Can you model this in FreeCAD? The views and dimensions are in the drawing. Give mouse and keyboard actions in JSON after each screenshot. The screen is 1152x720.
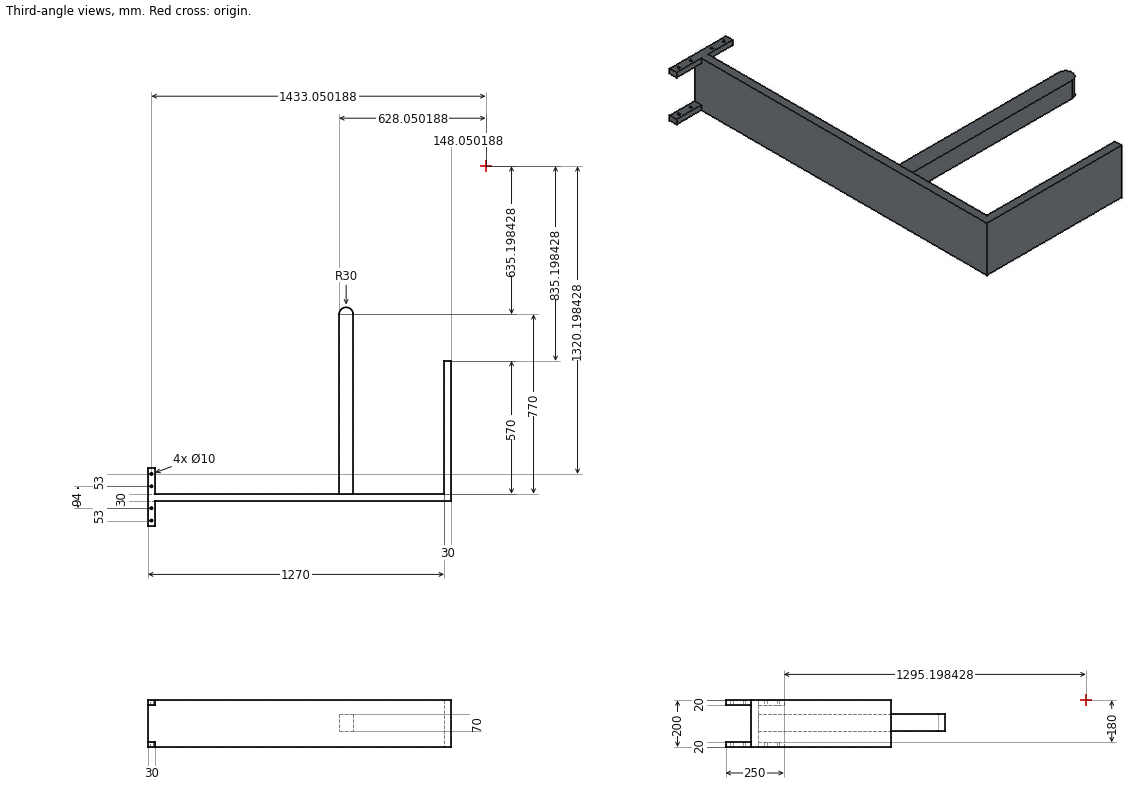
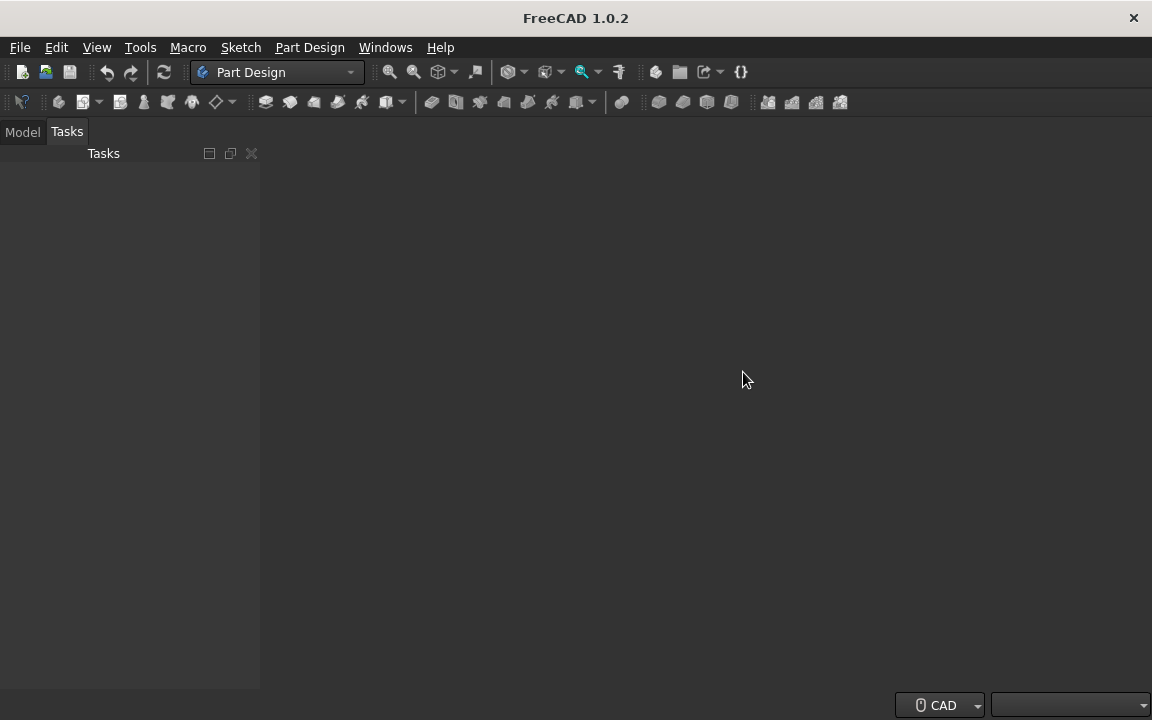
{"action": "left_click", "coordinate": [22, 72]}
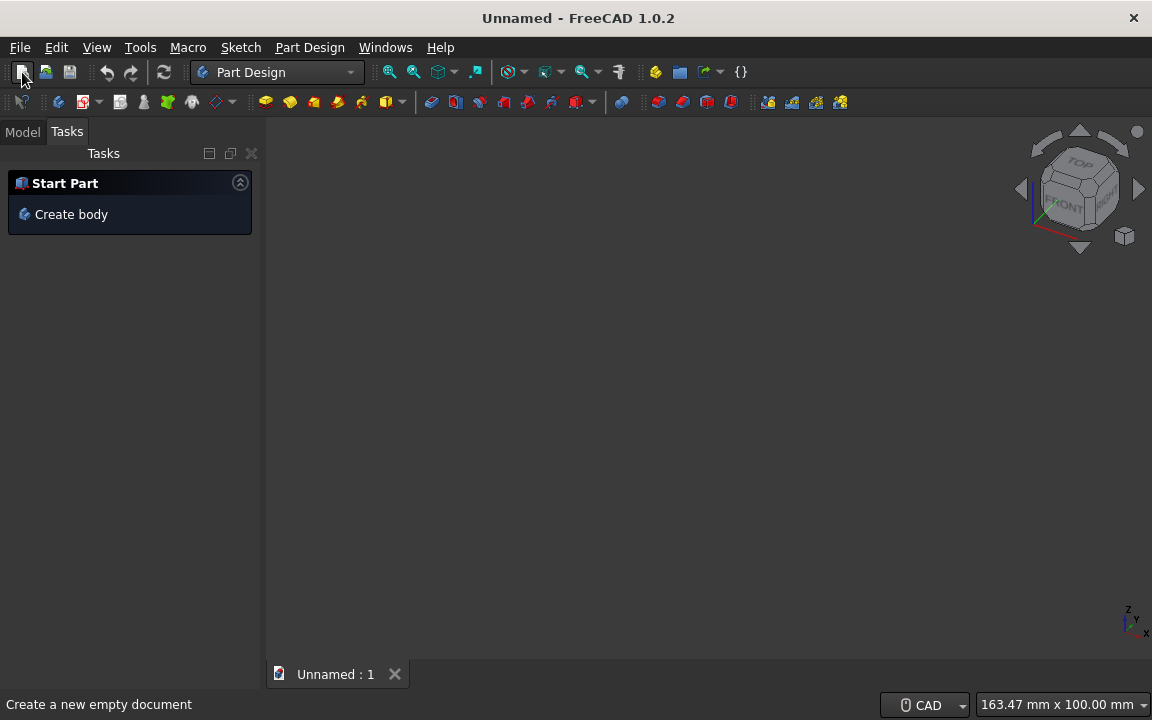
{"action": "left_click", "coordinate": [84, 102]}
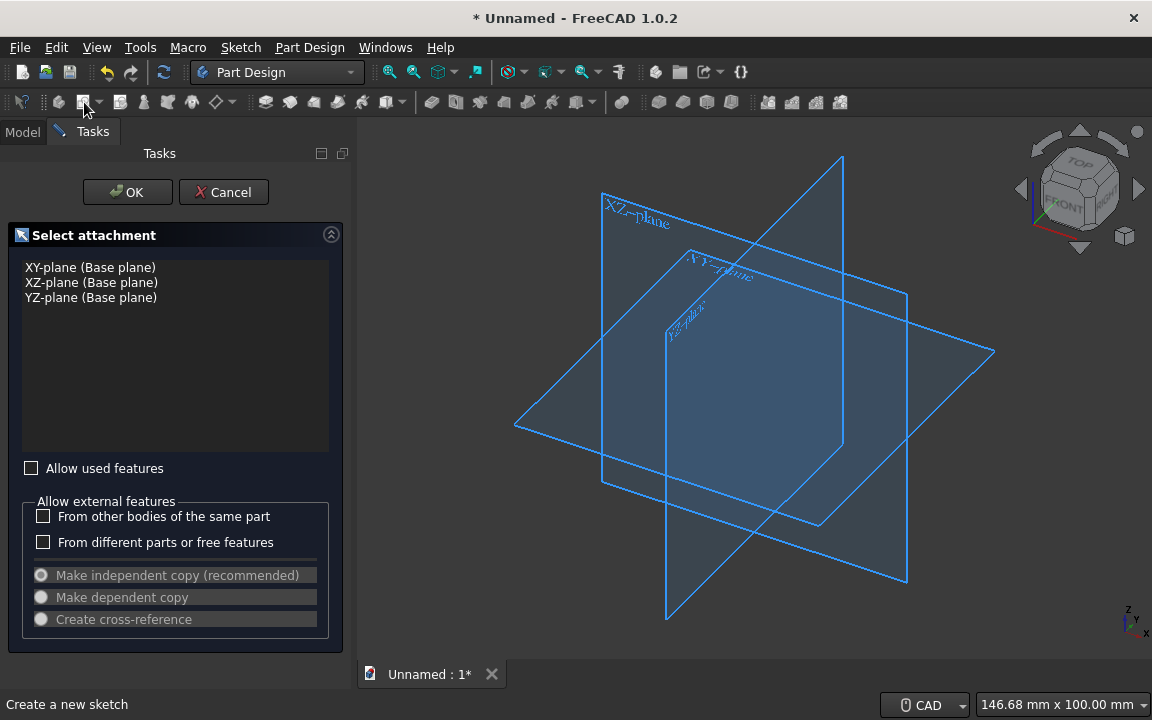
{"action": "left_click", "coordinate": [82, 268]}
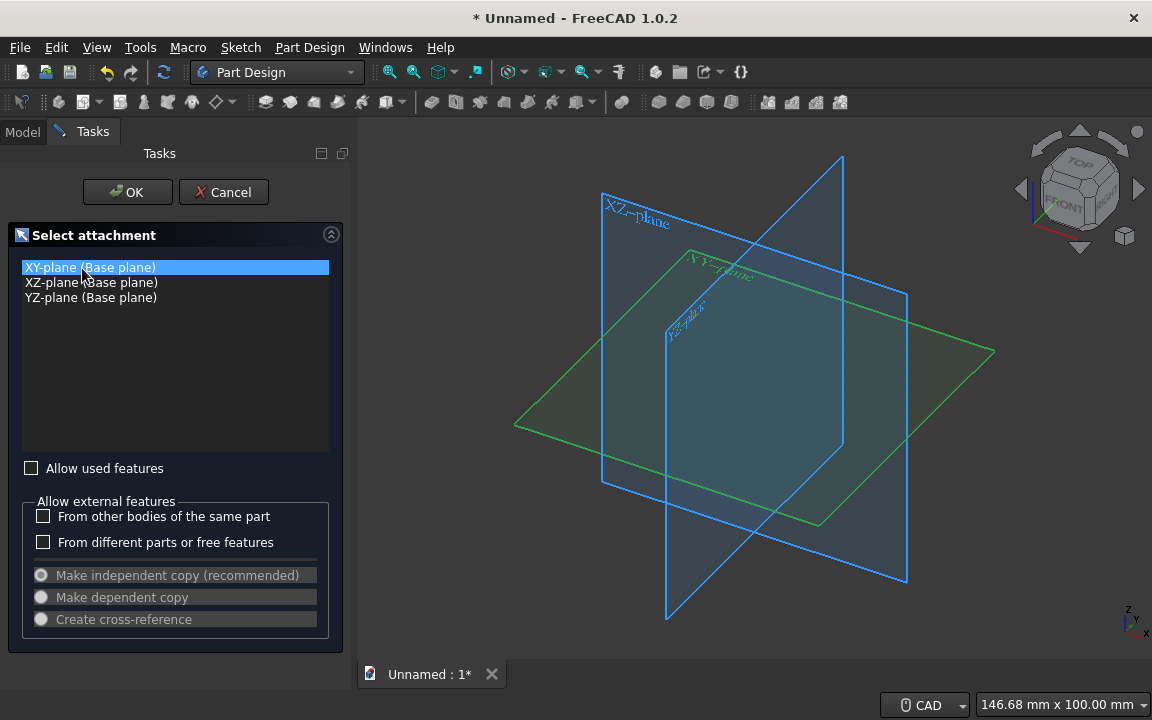
{"action": "left_click", "coordinate": [128, 192]}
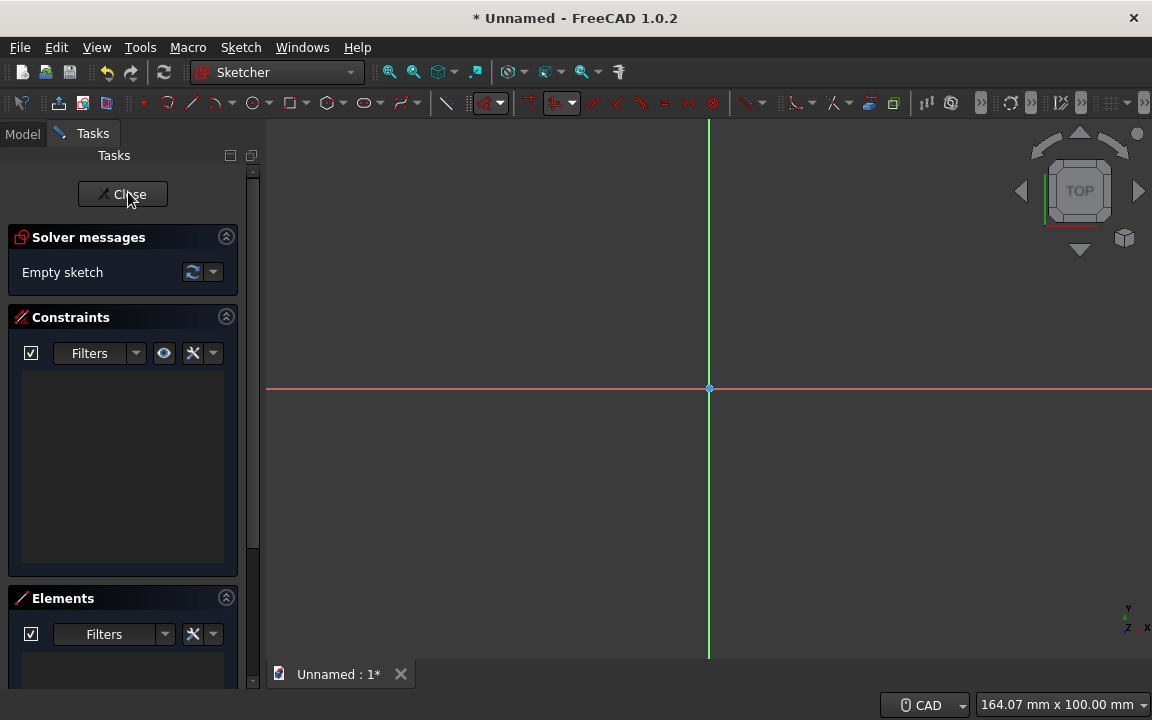
{"action": "scroll", "coordinate": [842, 186], "scroll_direction": "down", "scroll_amount": 15}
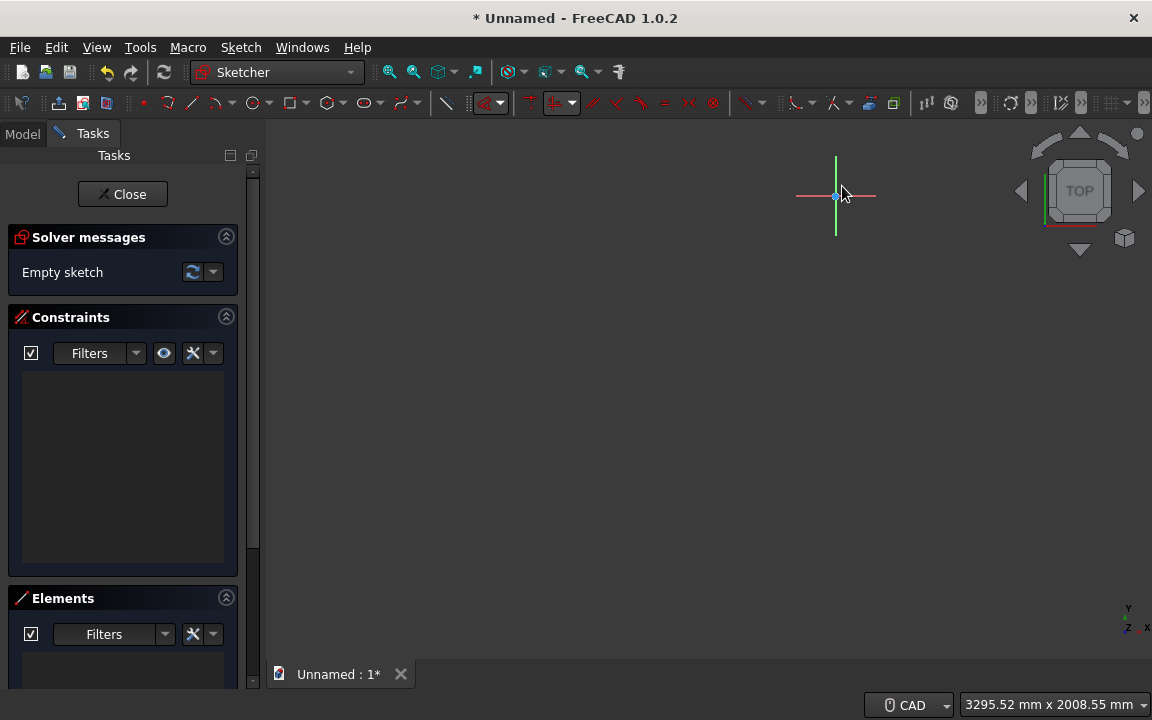
{"action": "left_click", "coordinate": [168, 104]}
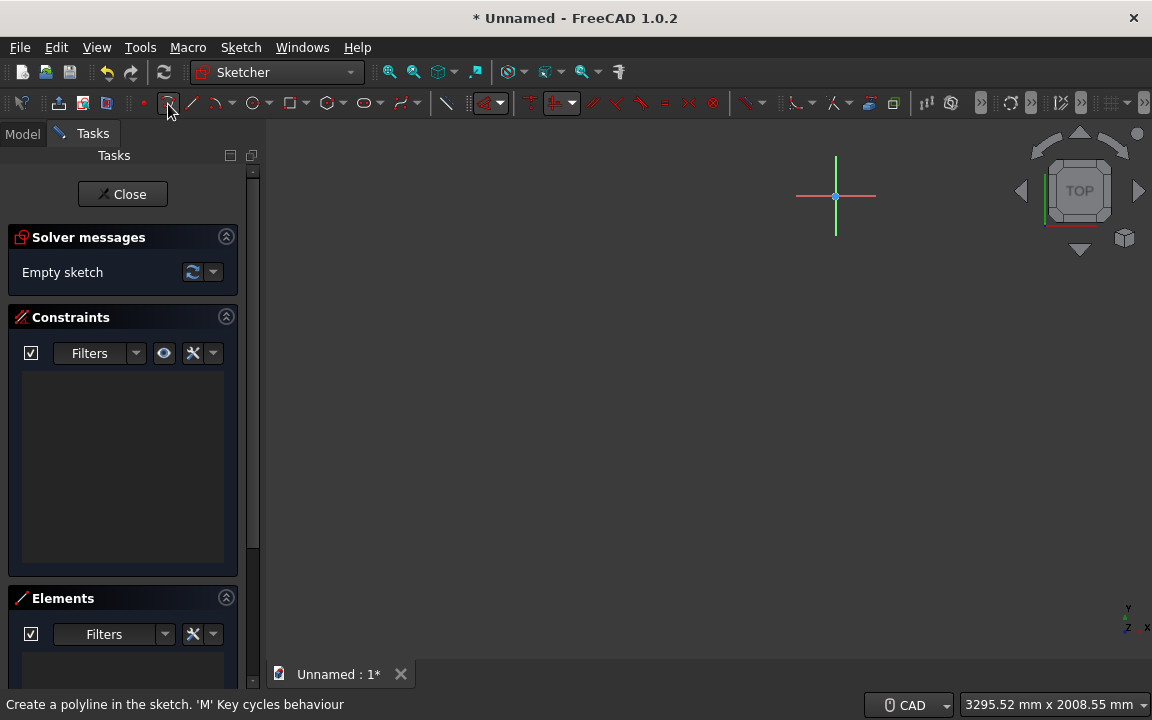
{"action": "left_click", "coordinate": [796, 421]}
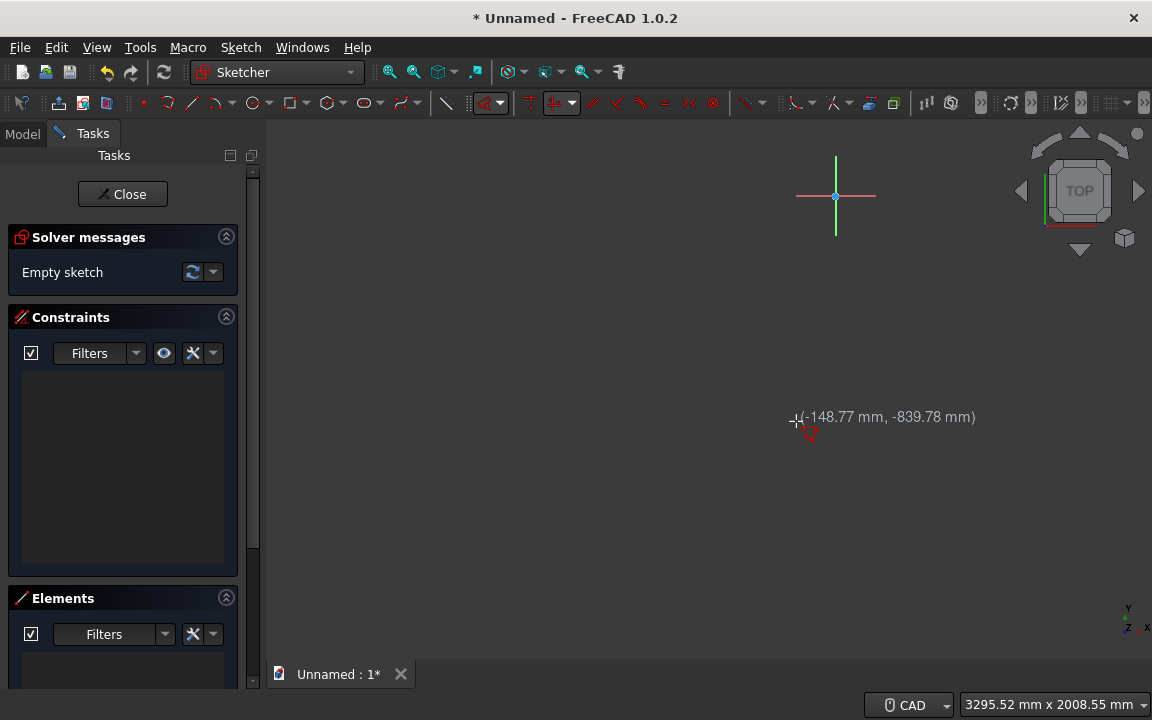
{"action": "scroll", "coordinate": [788, 421], "scroll_direction": "up", "scroll_amount": 4}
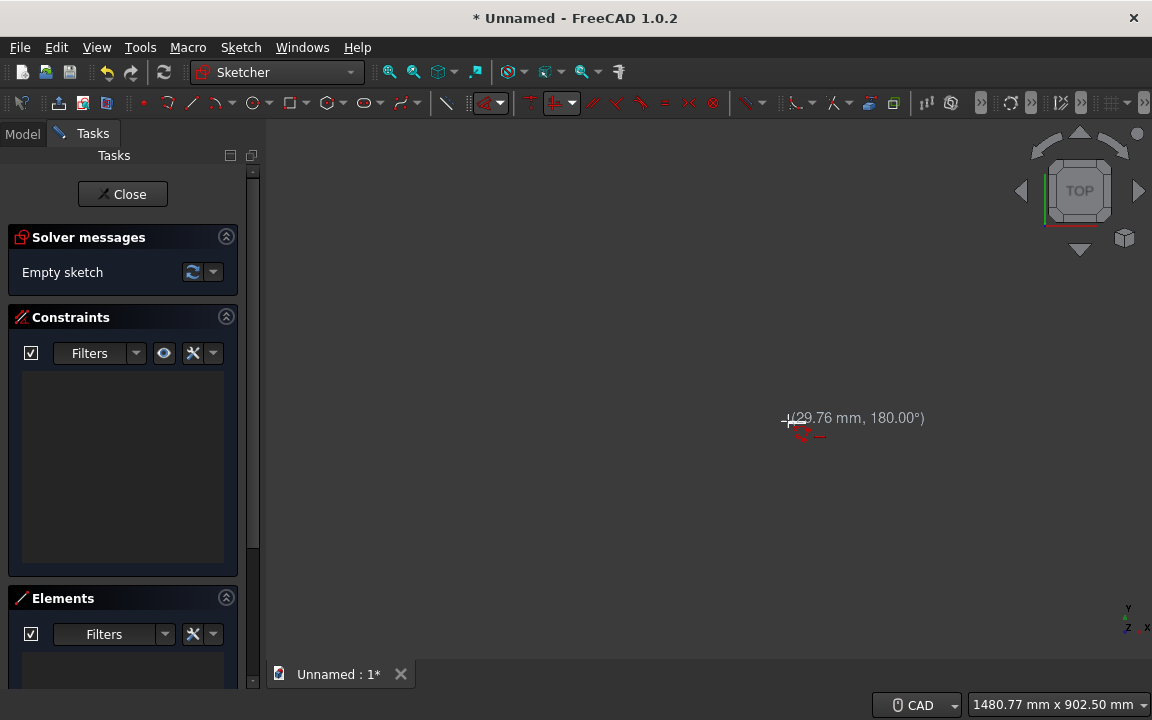
{"action": "left_click", "coordinate": [788, 420]}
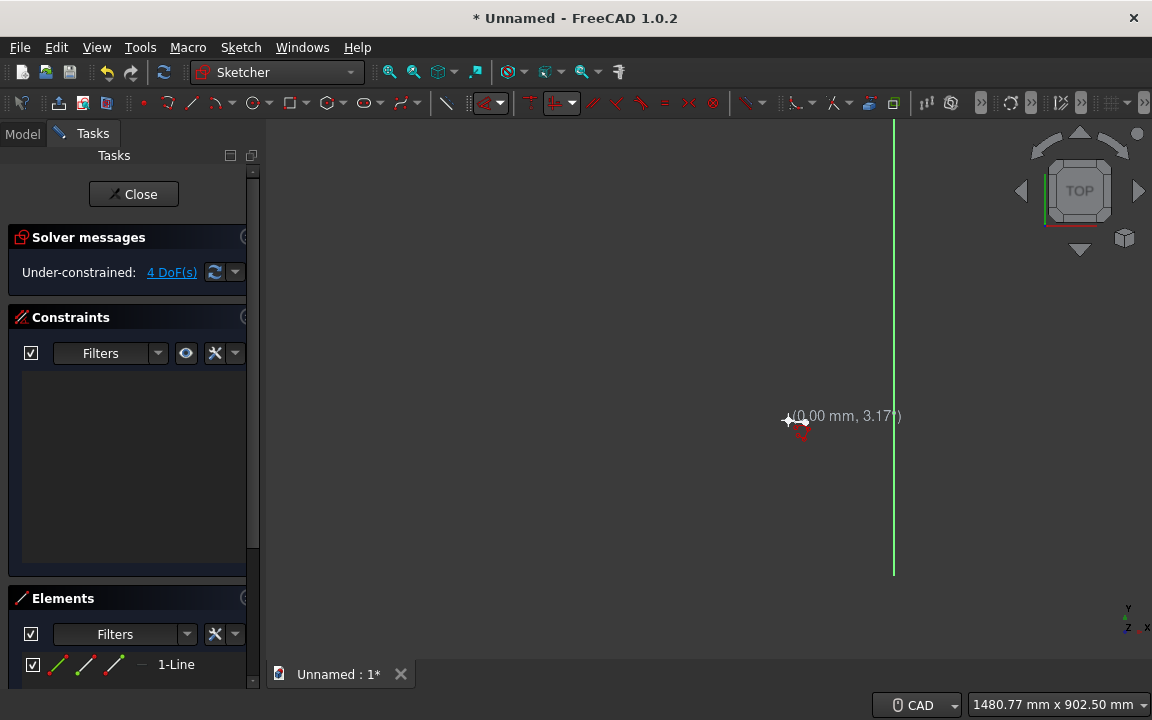
{"action": "scroll", "coordinate": [745, 412], "scroll_direction": "down", "scroll_amount": 5}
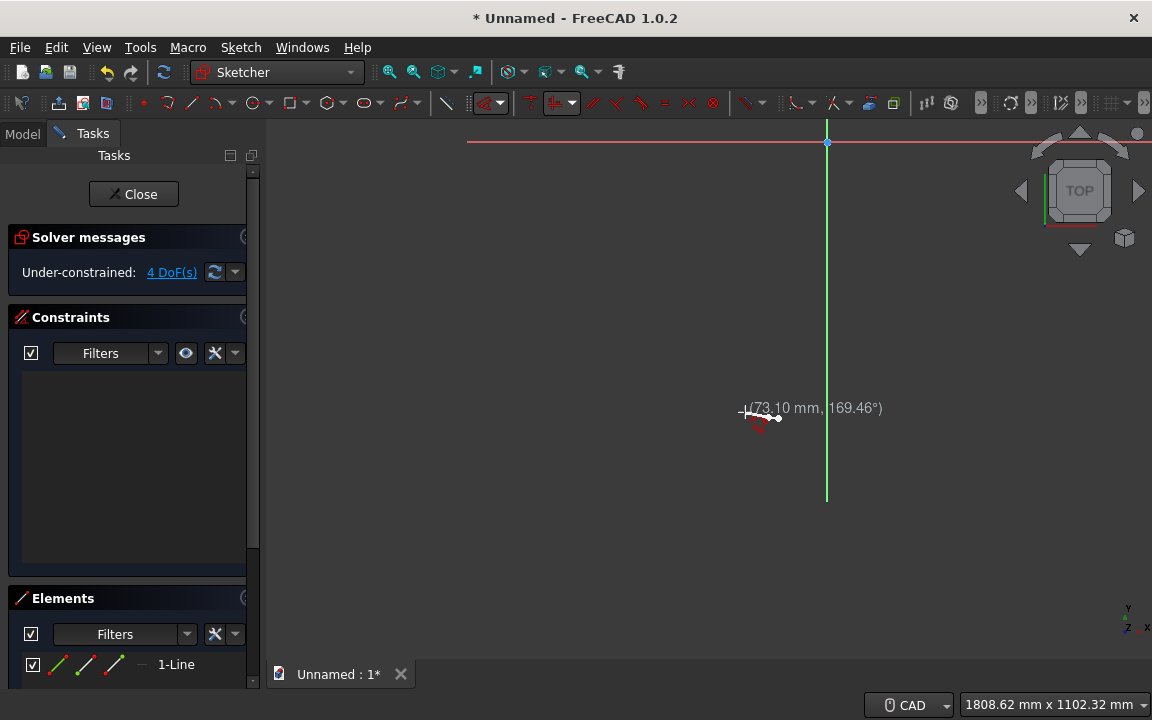
{"action": "left_click", "coordinate": [761, 541]}
{"action": "left_click", "coordinate": [481, 541]}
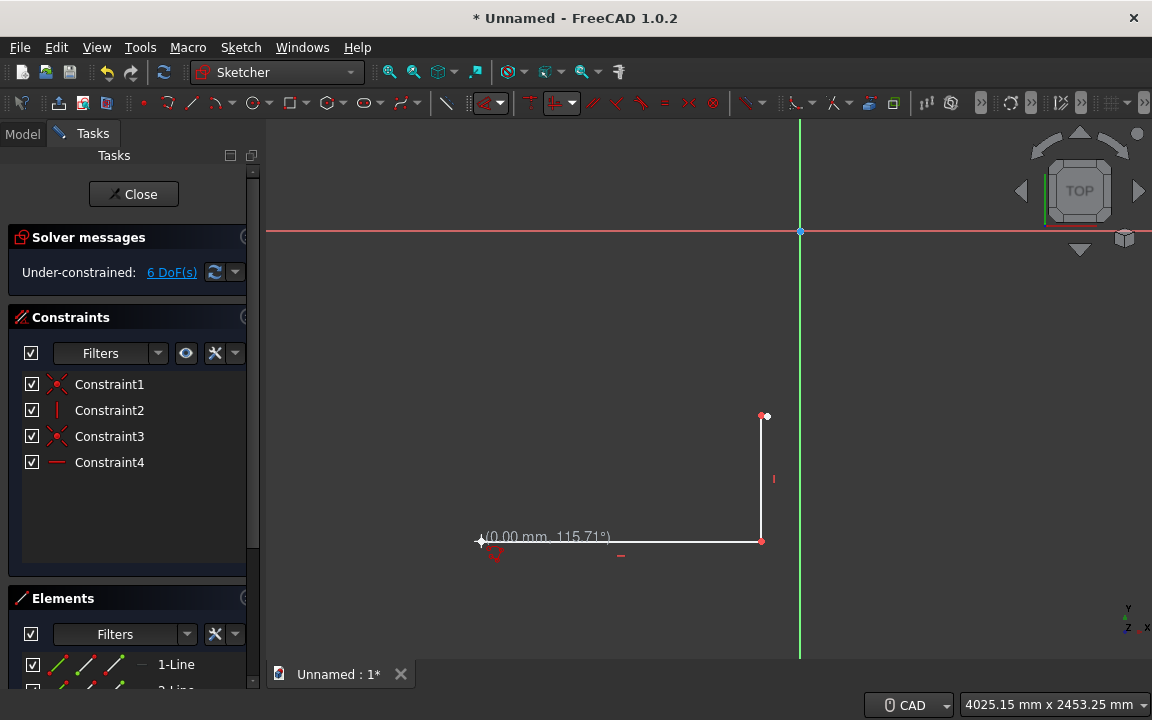
{"action": "scroll", "coordinate": [481, 547], "scroll_direction": "up", "scroll_amount": 5}